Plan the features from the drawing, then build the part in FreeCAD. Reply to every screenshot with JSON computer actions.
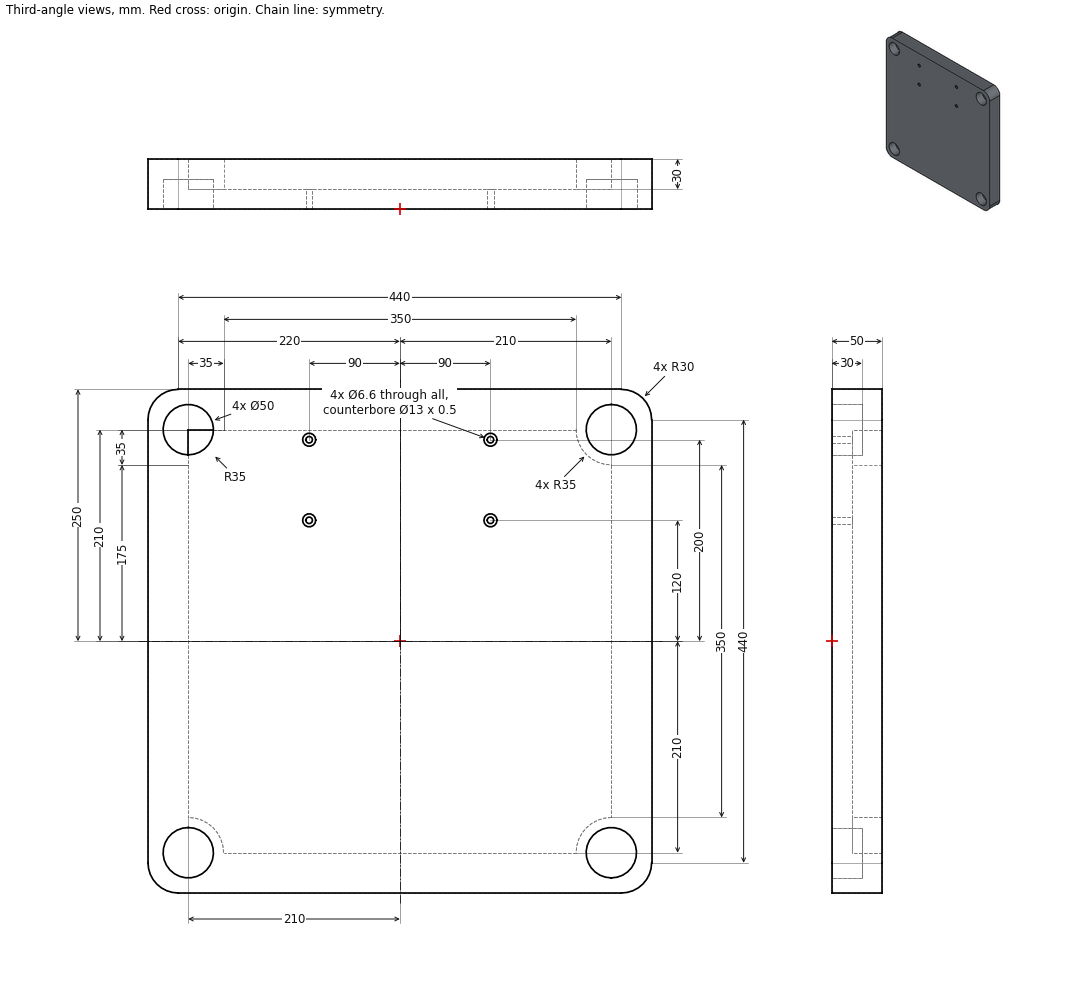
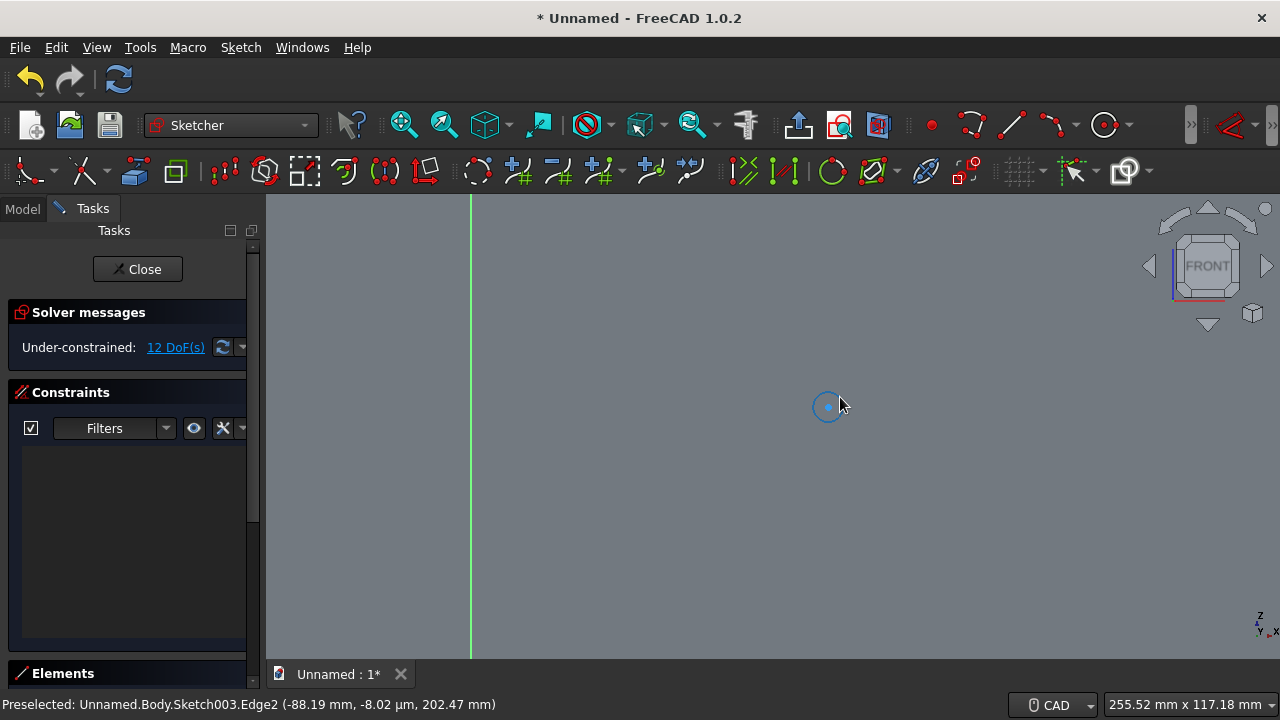
{"action": "left_click", "coordinate": [839, 397]}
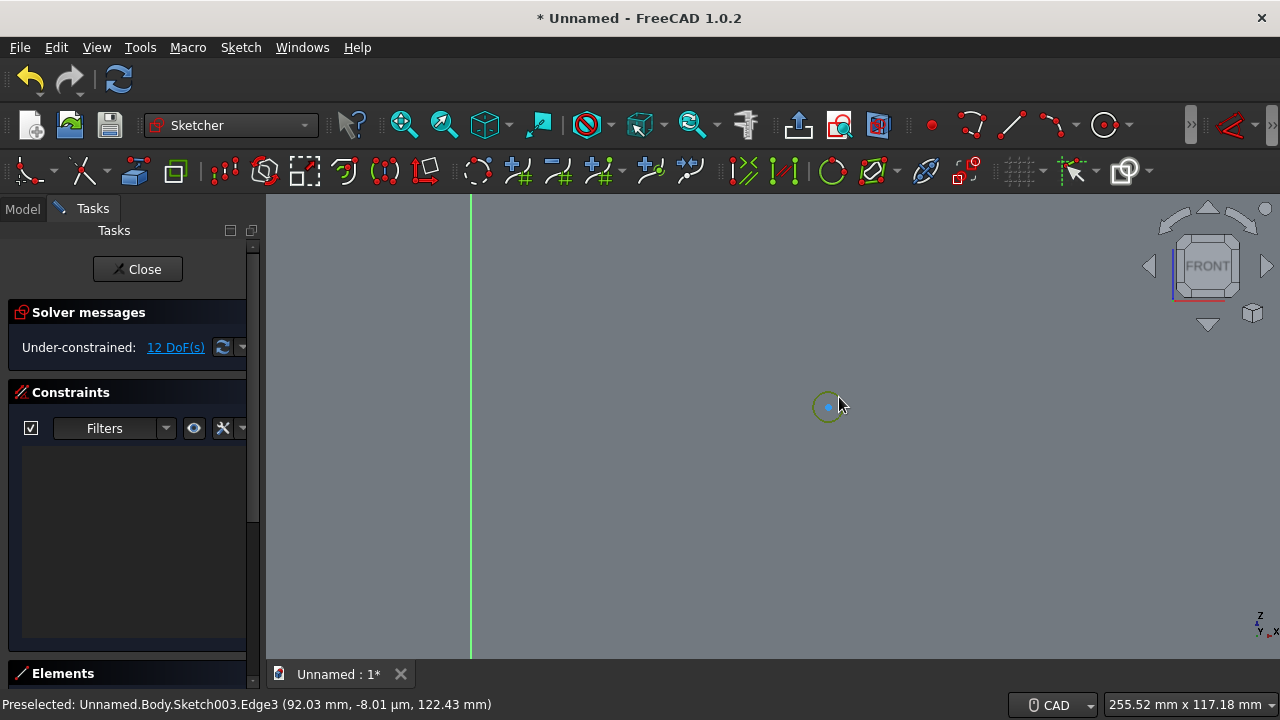
{"action": "scroll", "coordinate": [840, 397], "scroll_direction": "down", "scroll_amount": 5}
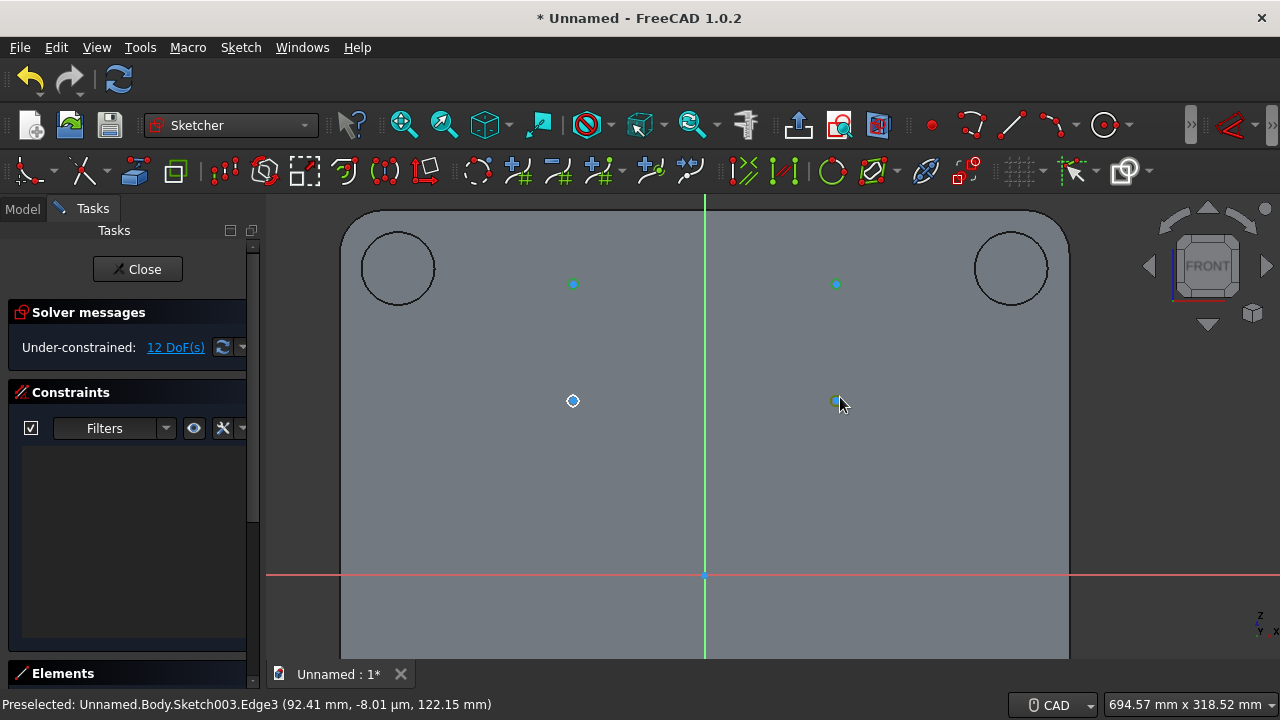
{"action": "scroll", "coordinate": [577, 397], "scroll_direction": "up", "scroll_amount": 5}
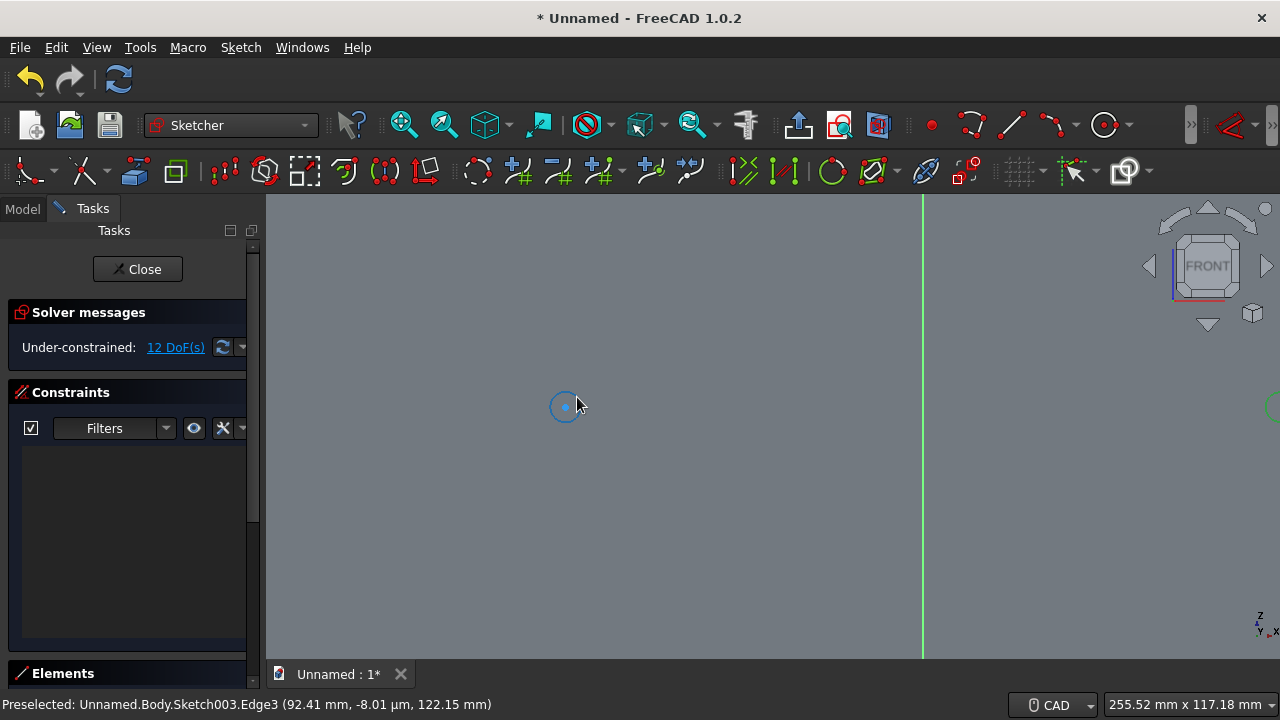
{"action": "left_click", "coordinate": [576, 396]}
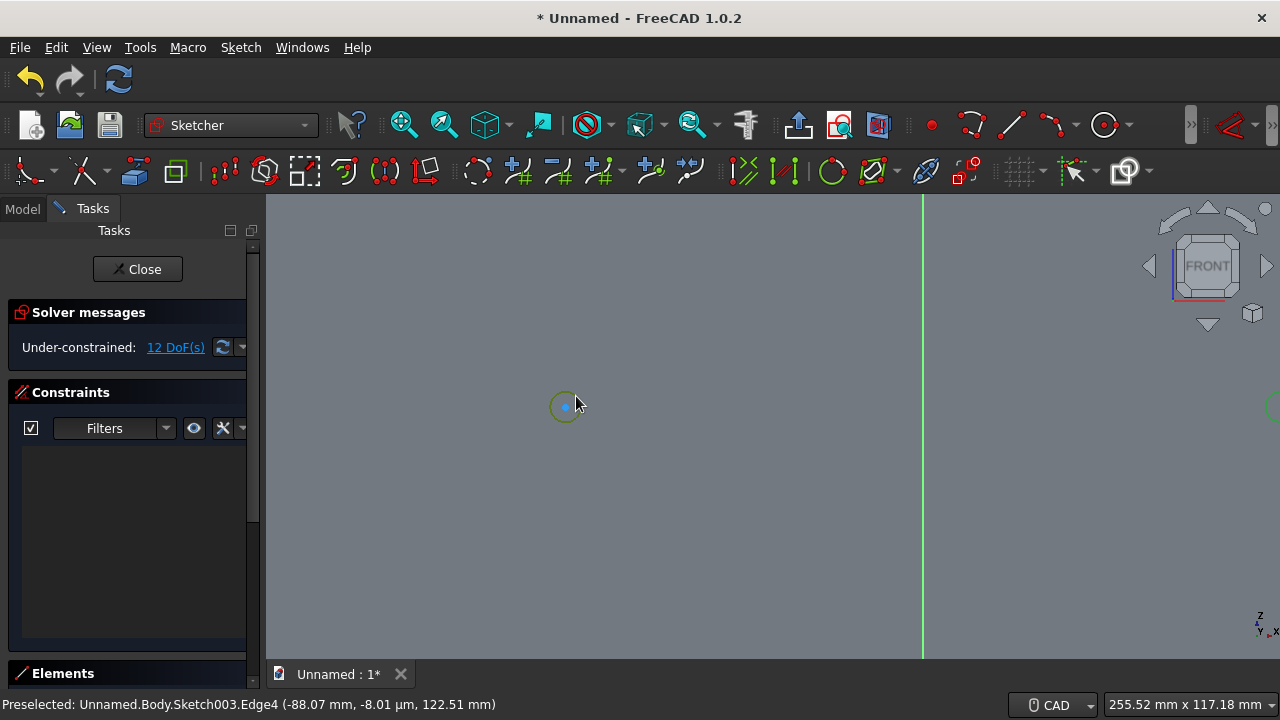
{"action": "key", "text": "e"}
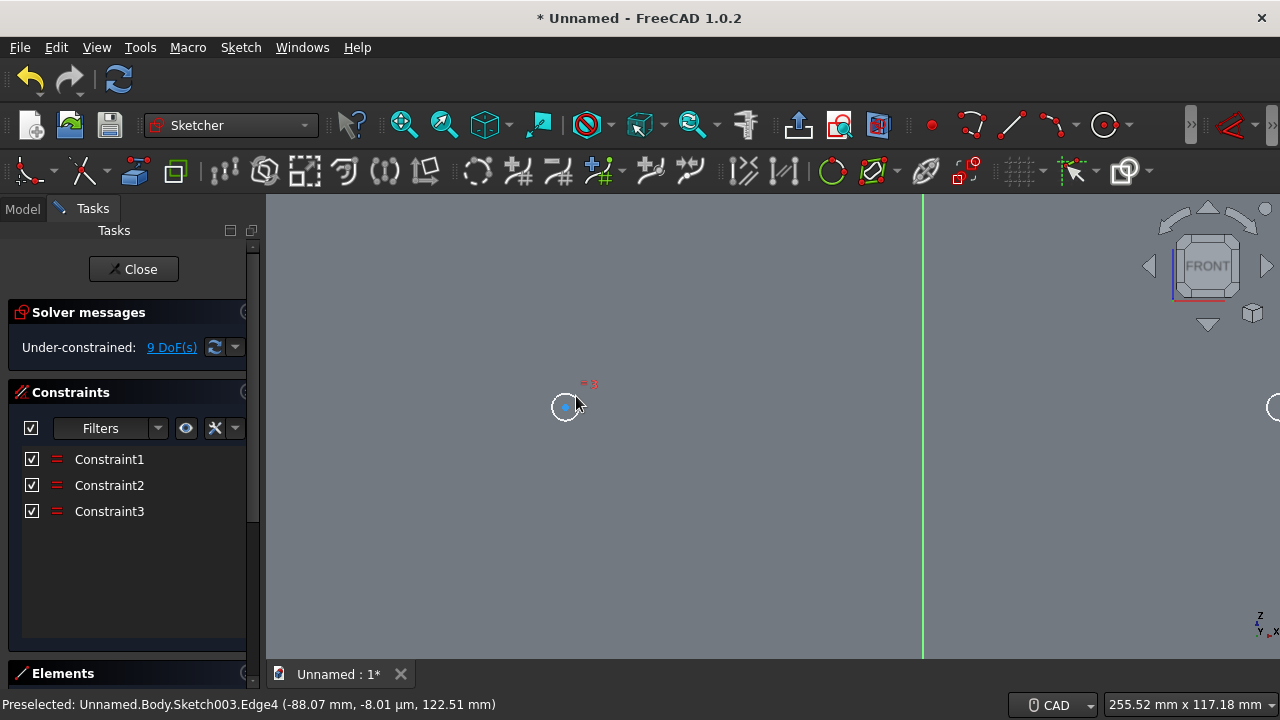
{"action": "scroll", "coordinate": [577, 397], "scroll_direction": "down", "scroll_amount": 5}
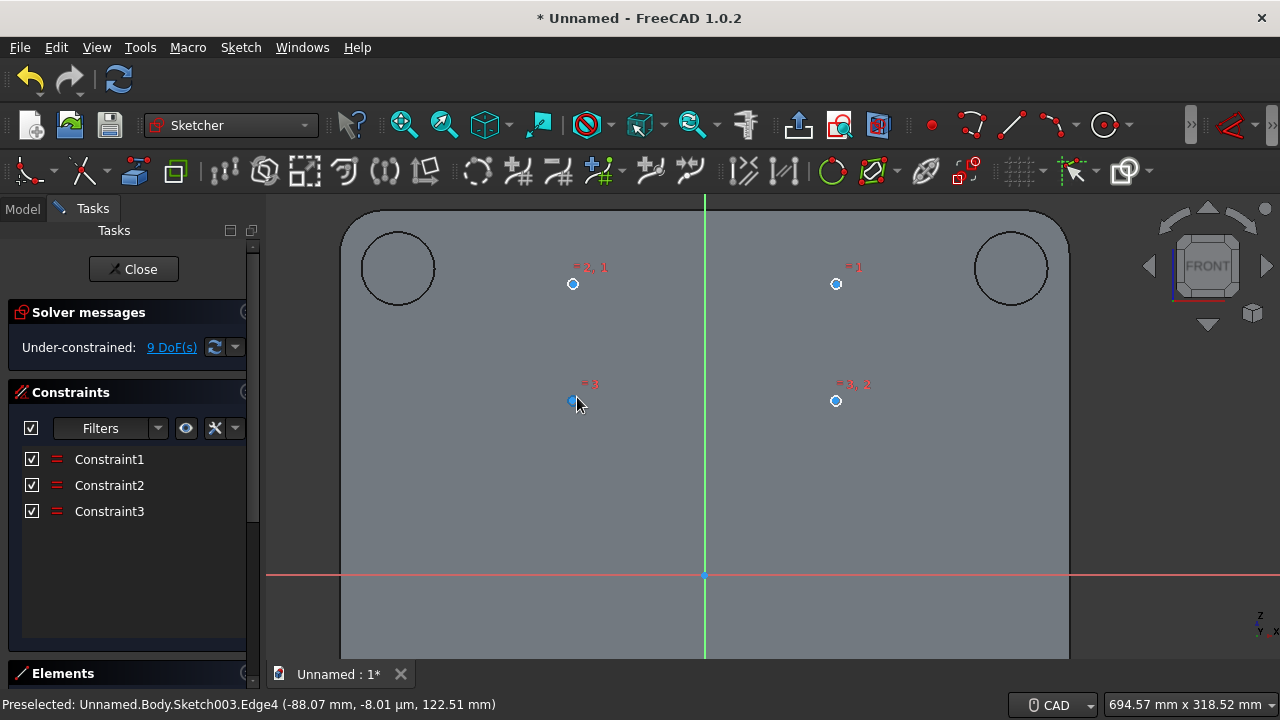
{"action": "left_click", "coordinate": [836, 284]}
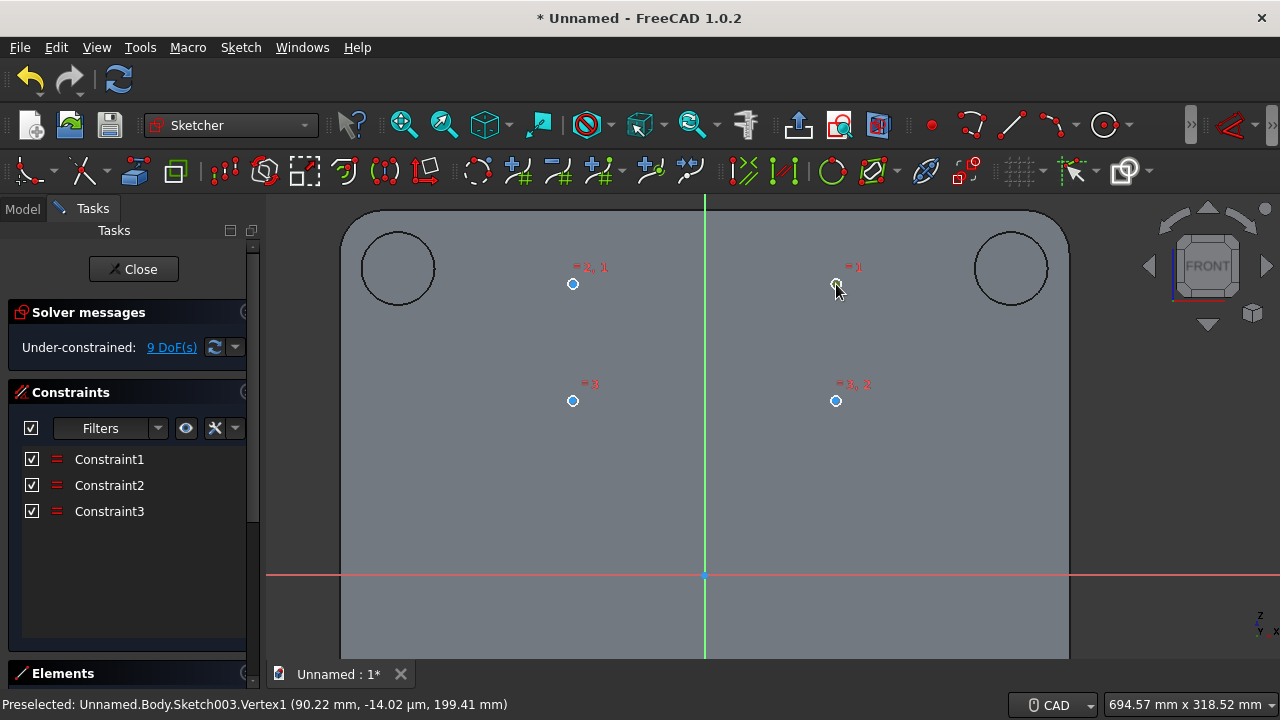
{"action": "left_click", "coordinate": [573, 284]}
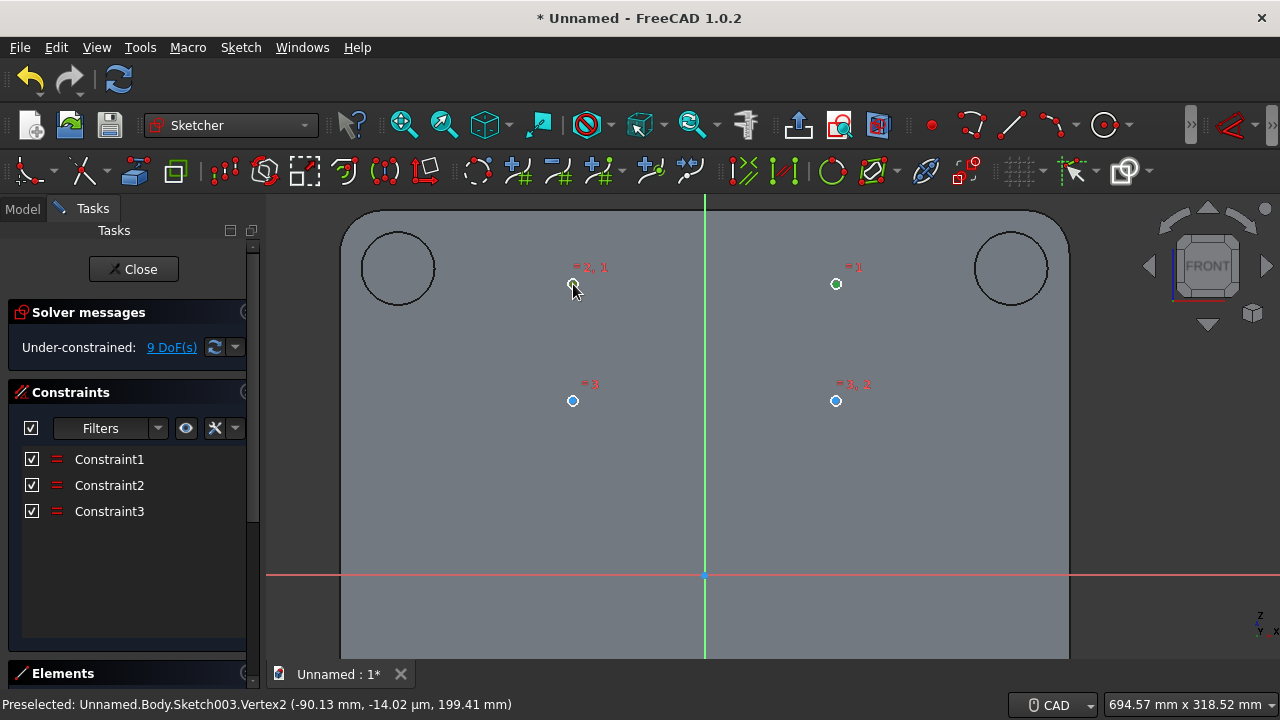
{"action": "key", "text": "h"}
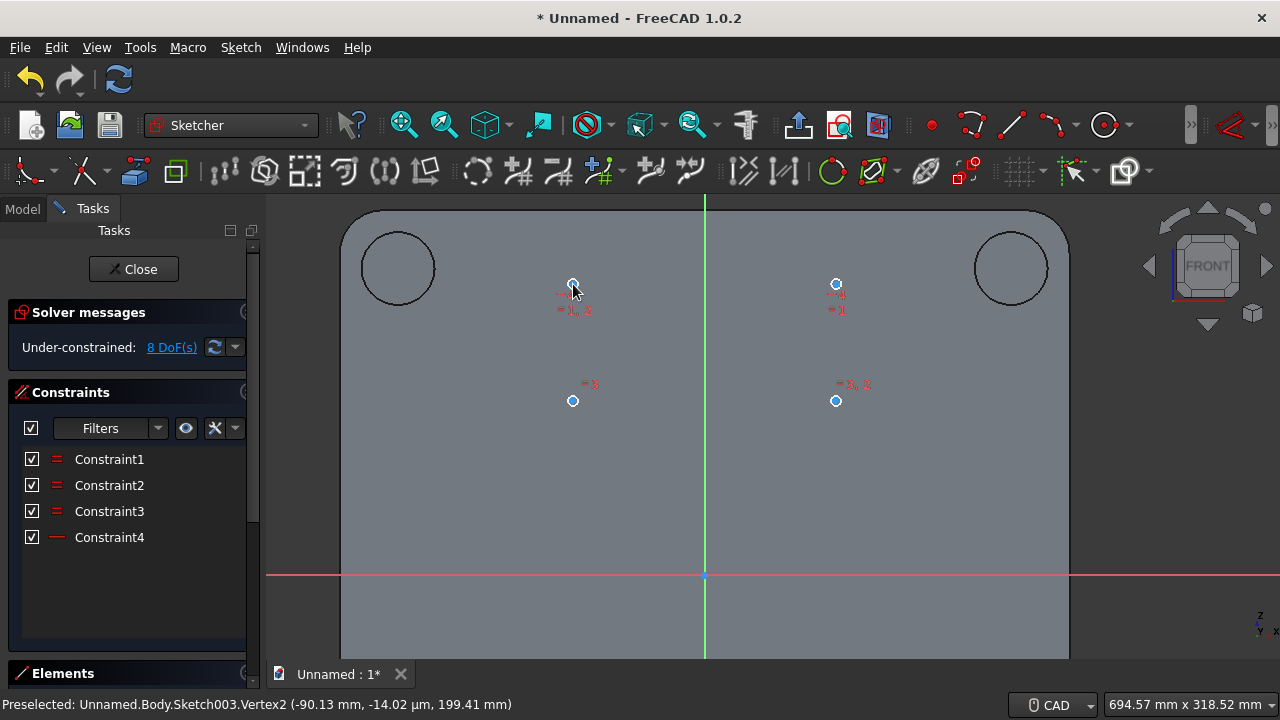
{"action": "left_click", "coordinate": [836, 284]}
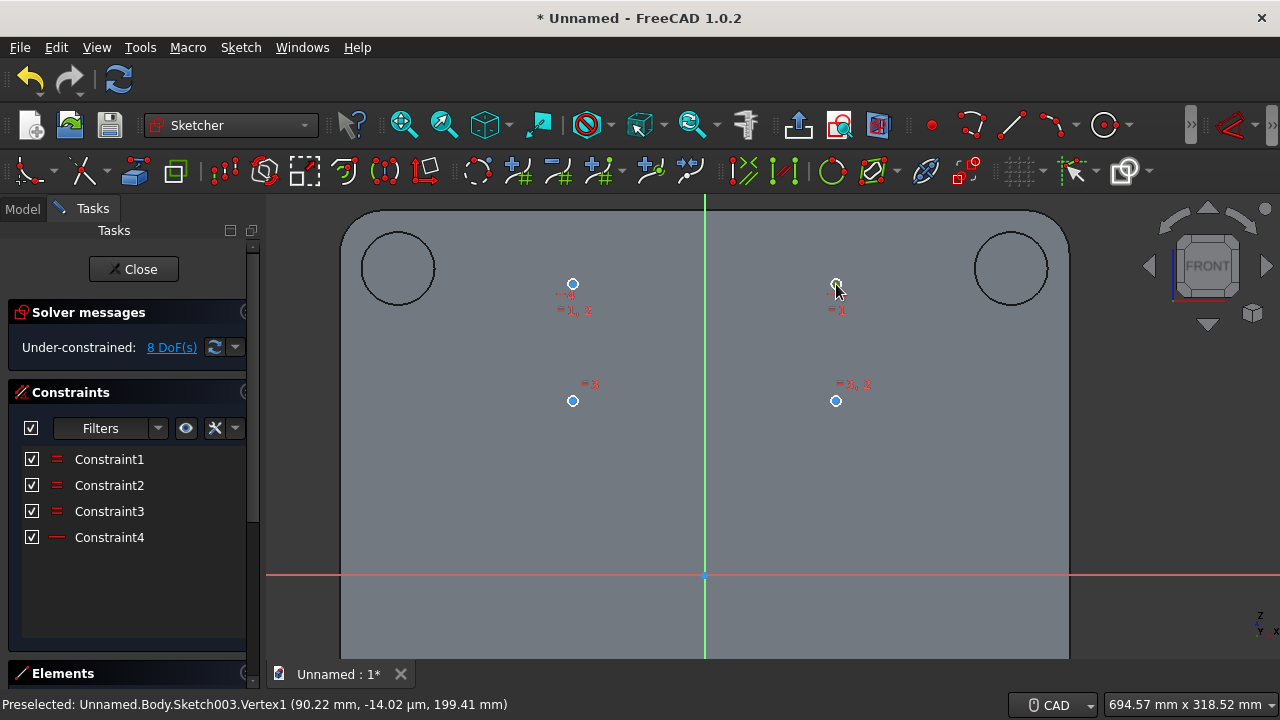
{"action": "left_click", "coordinate": [836, 401]}